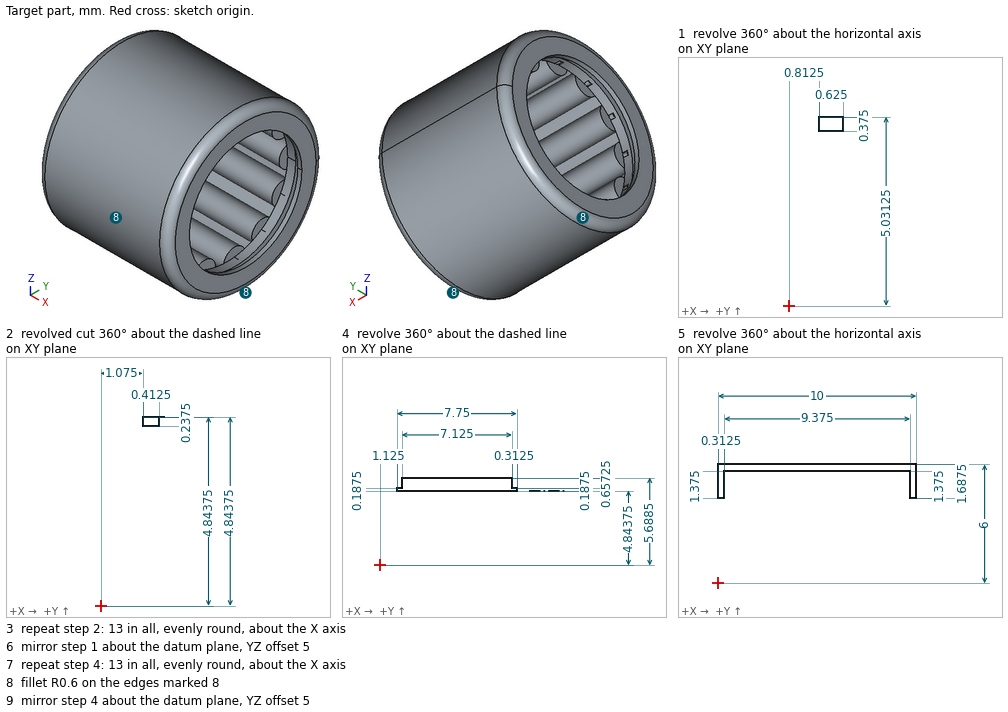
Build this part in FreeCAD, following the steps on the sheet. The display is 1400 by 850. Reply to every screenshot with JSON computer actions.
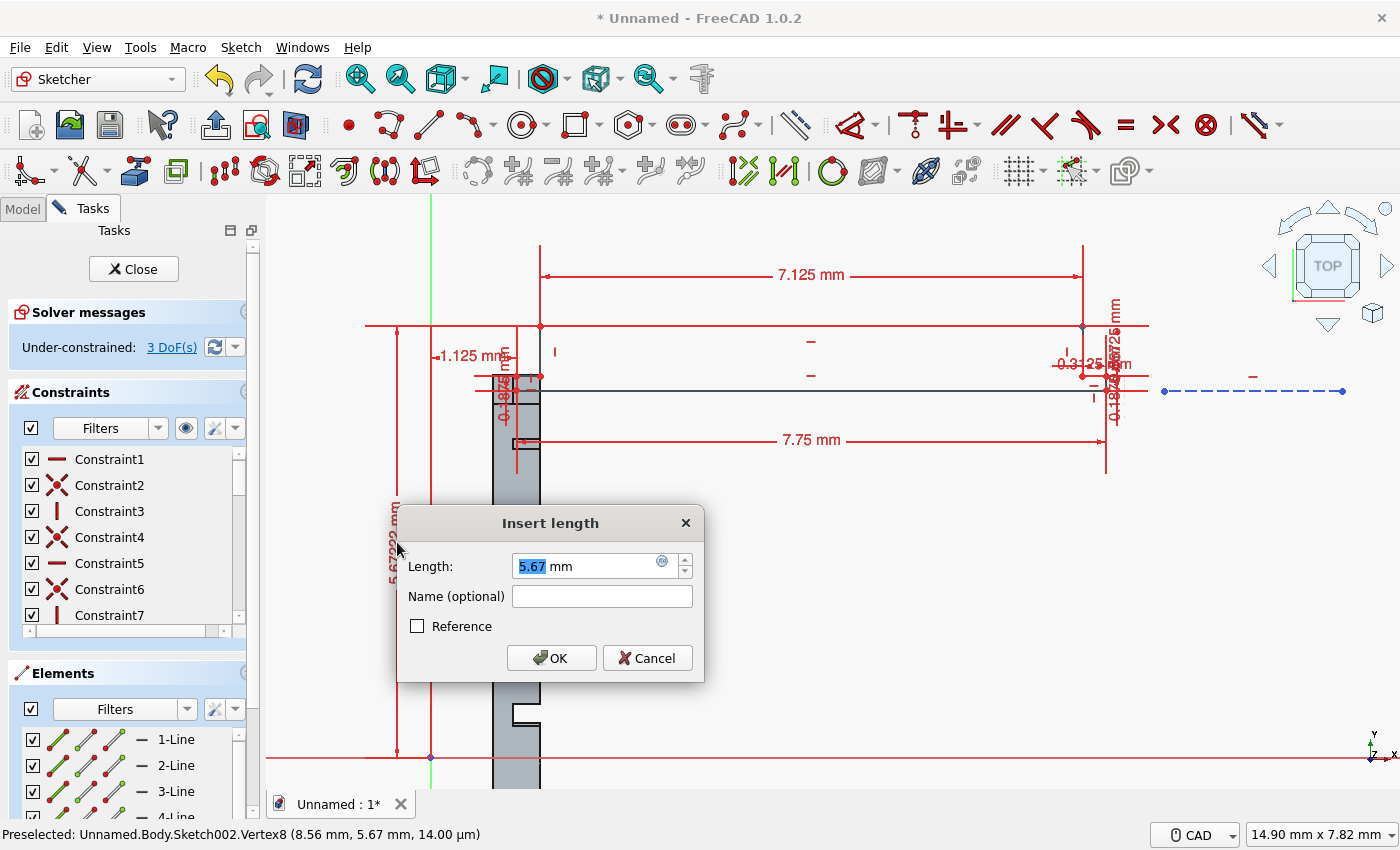
{"action": "type", "text": "5.6885"}
{"action": "key", "text": "Return"}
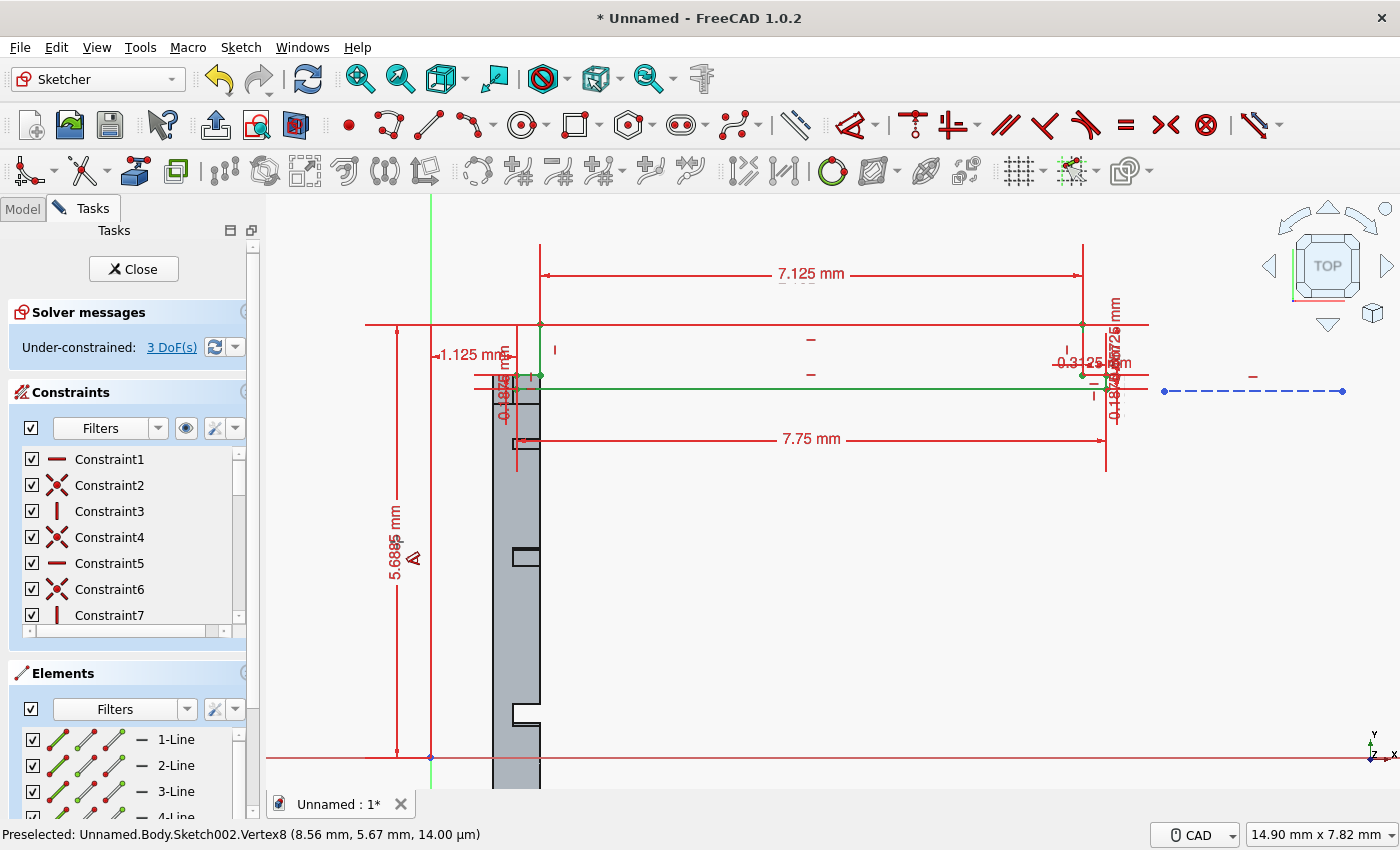
{"action": "left_click", "coordinate": [1165, 391]}
{"action": "left_click", "coordinate": [397, 575]}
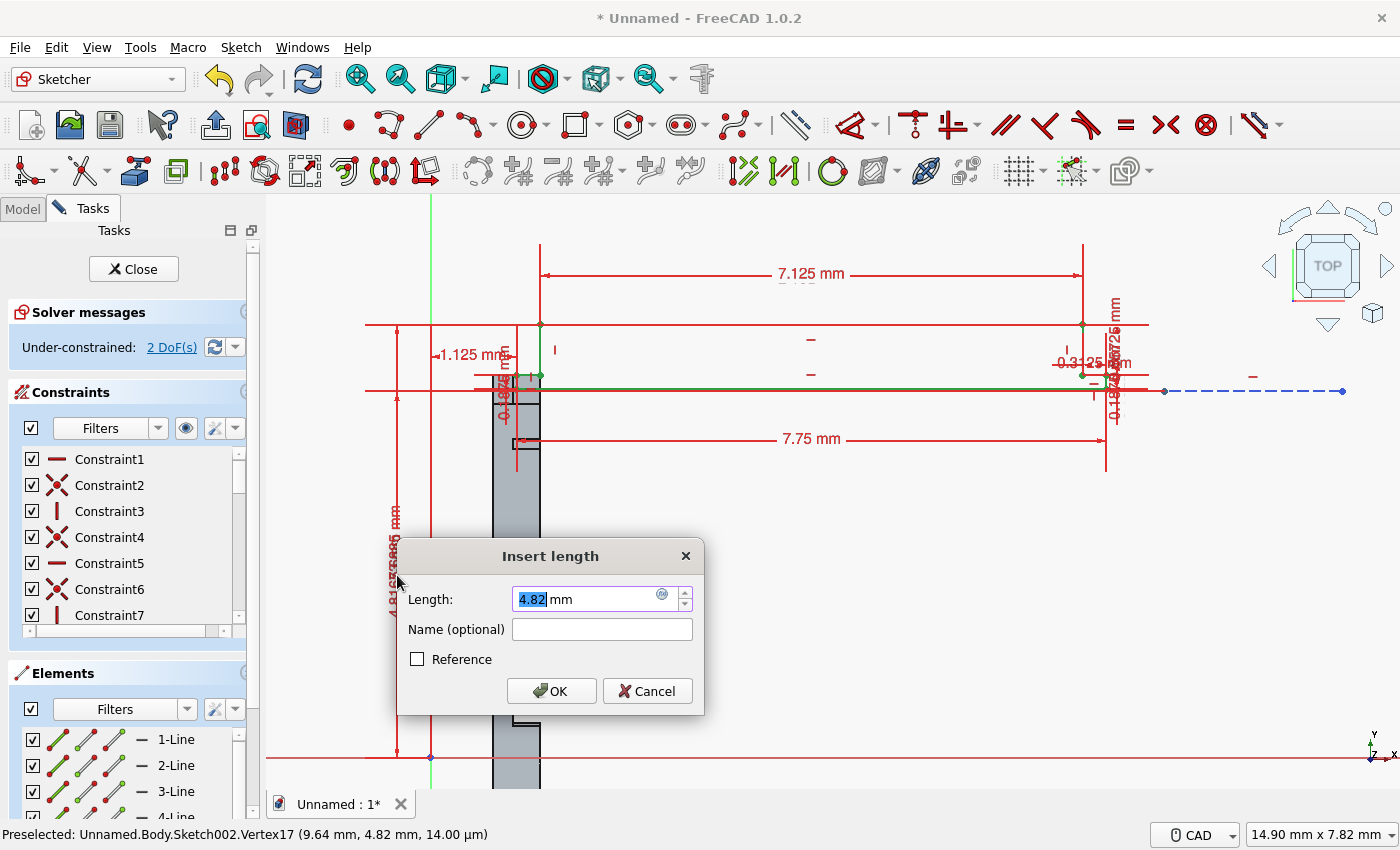
{"action": "type", "text": "4.84375"}
{"action": "key", "text": "Return"}
{"action": "key", "text": "Escape"}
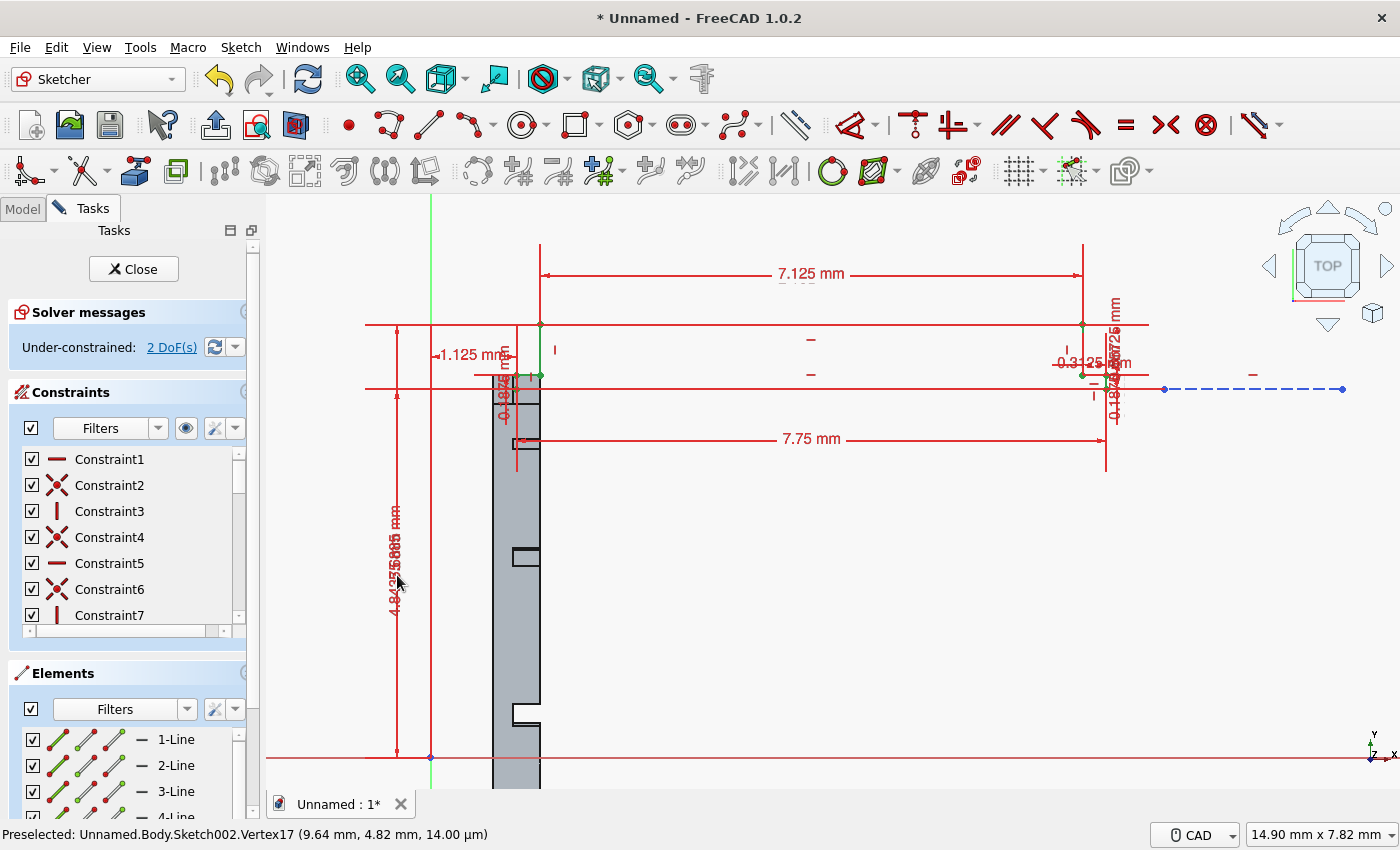
{"action": "left_click", "coordinate": [134, 269]}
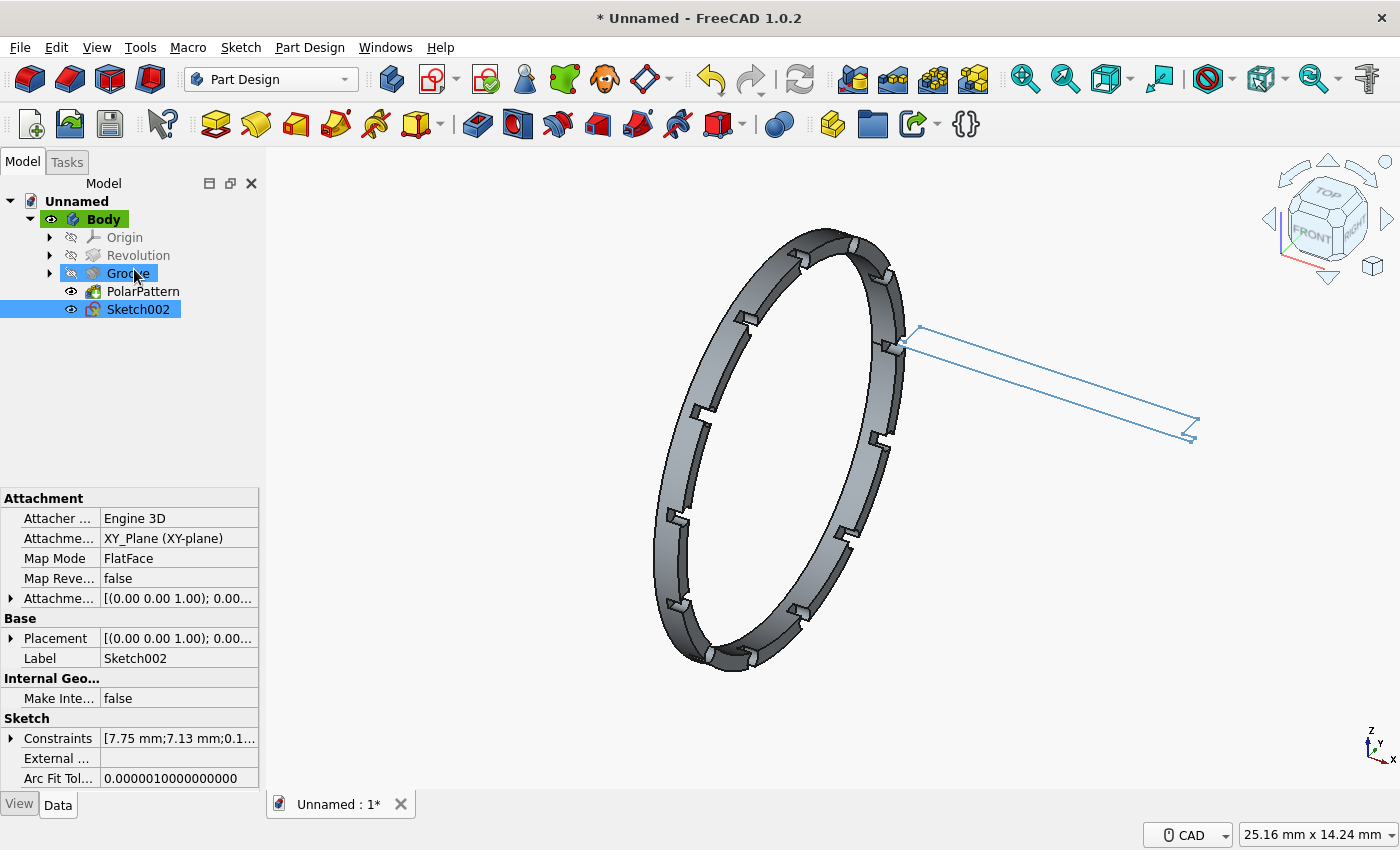
{"action": "left_click", "coordinate": [256, 124]}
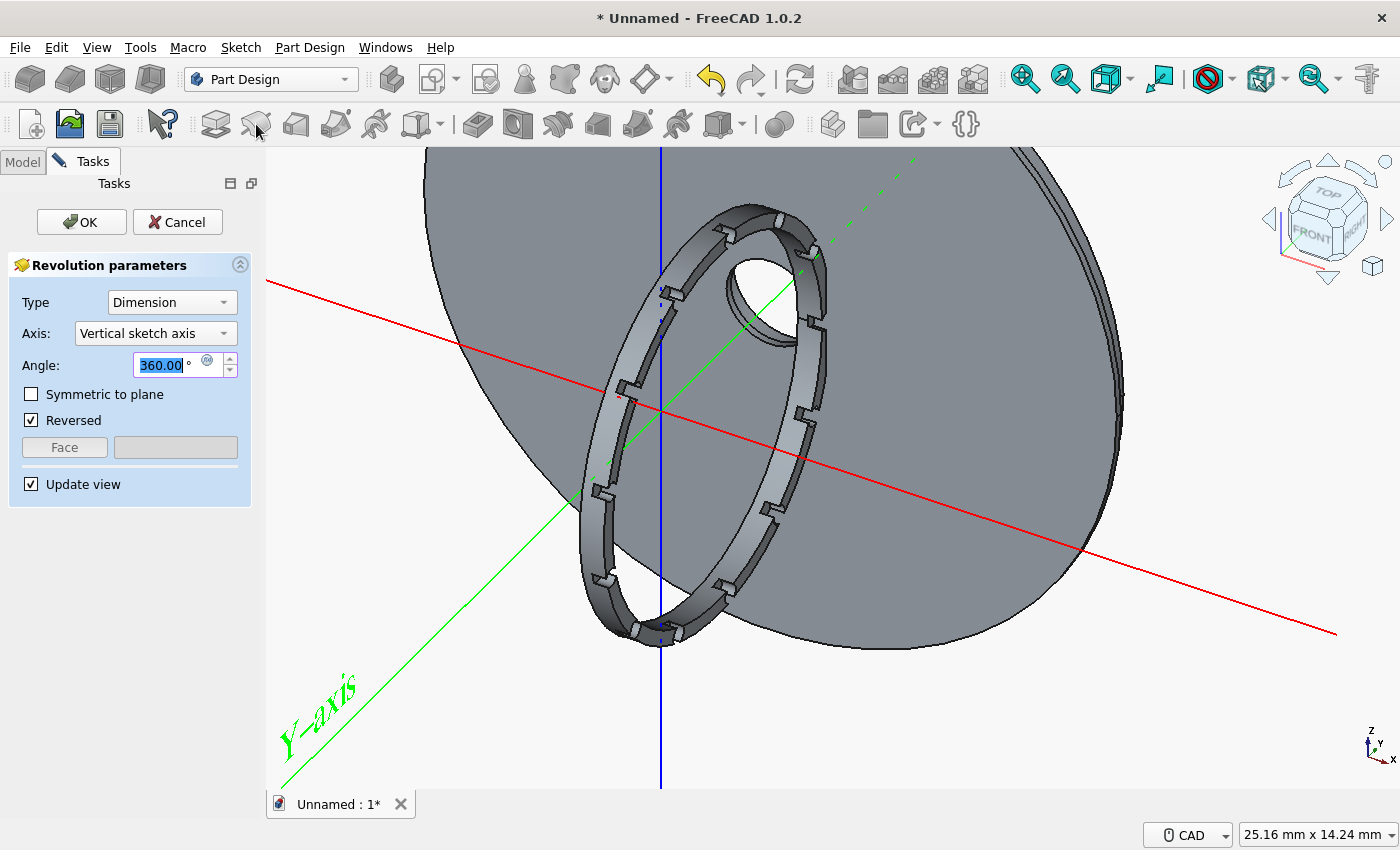
{"action": "left_click", "coordinate": [156, 334]}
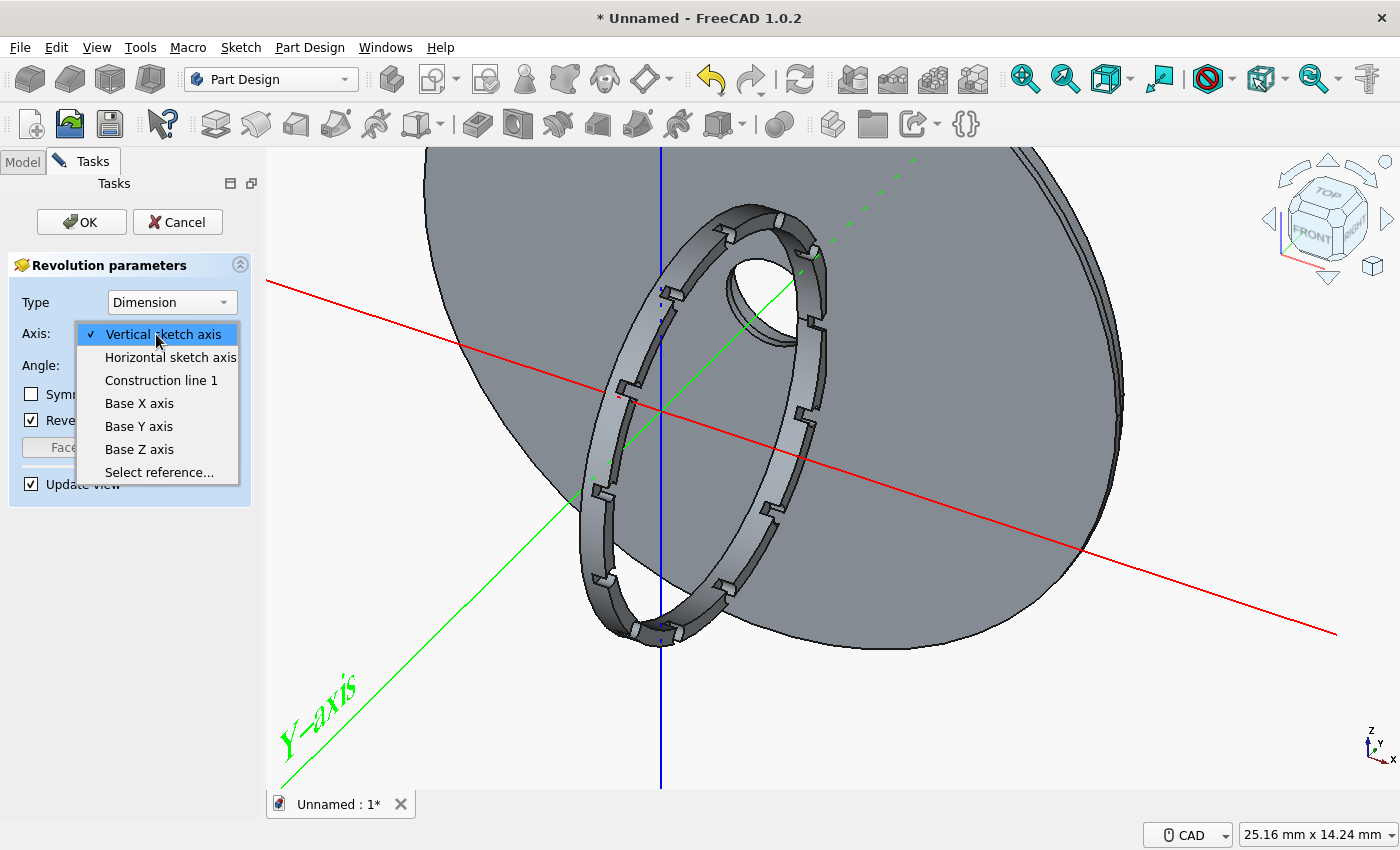
{"action": "left_click", "coordinate": [156, 380]}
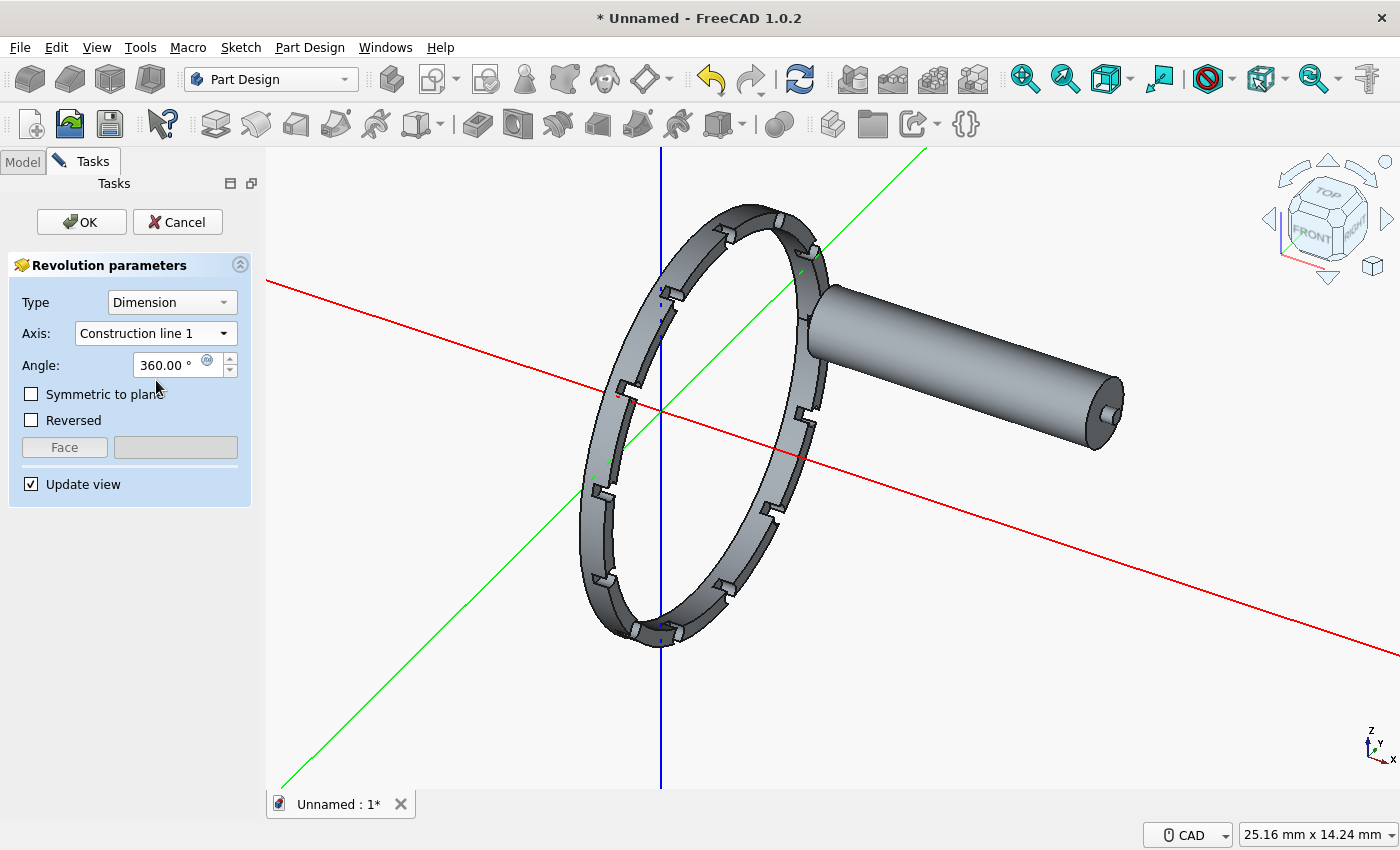
{"action": "left_click", "coordinate": [82, 222]}